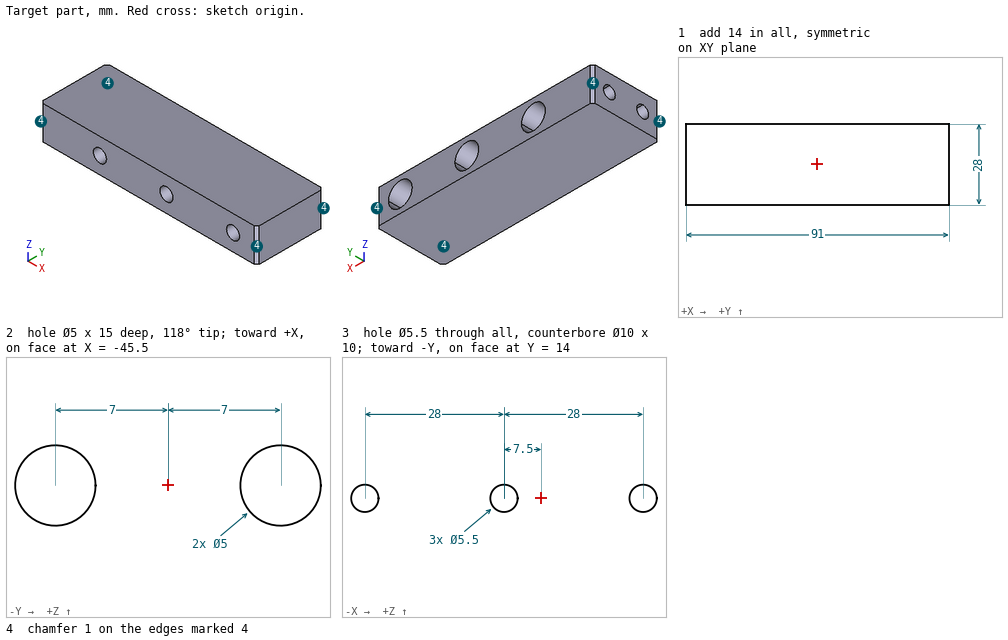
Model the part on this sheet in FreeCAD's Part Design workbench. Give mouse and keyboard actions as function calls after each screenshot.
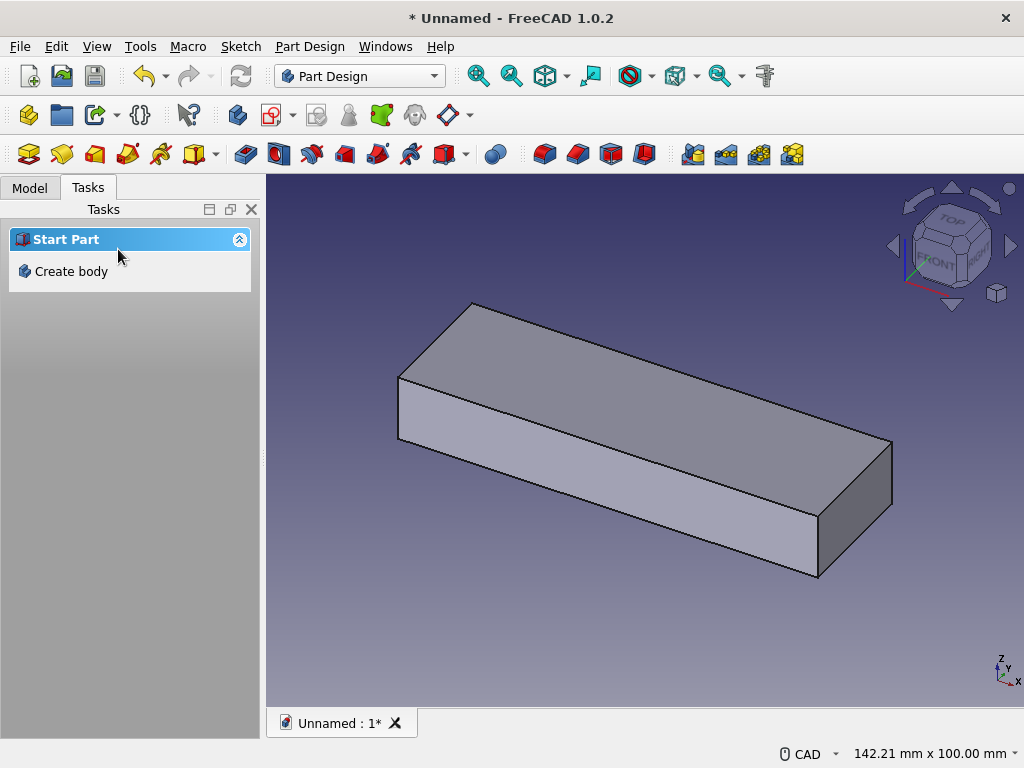
key(6)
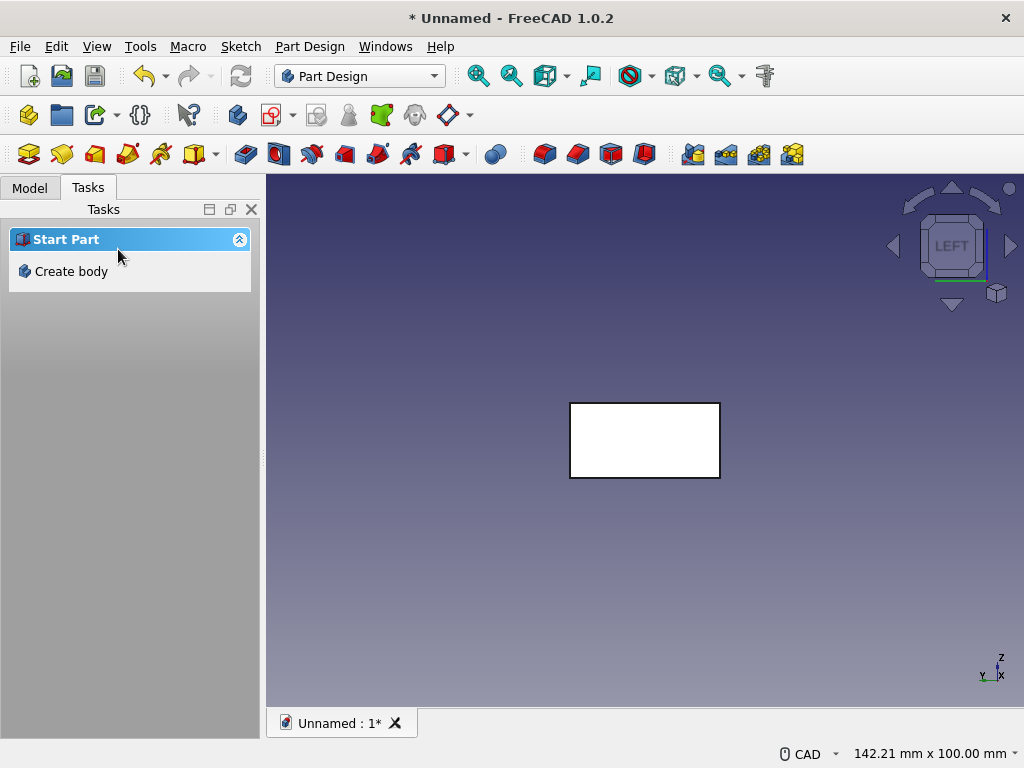
click(479, 76)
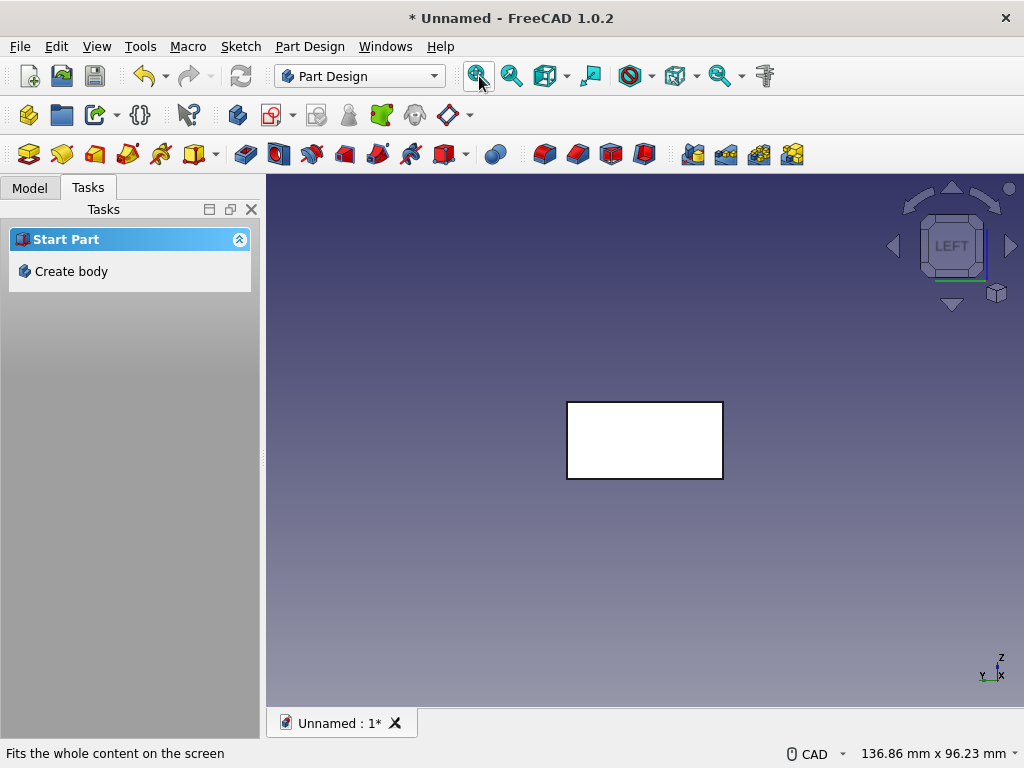
click(623, 439)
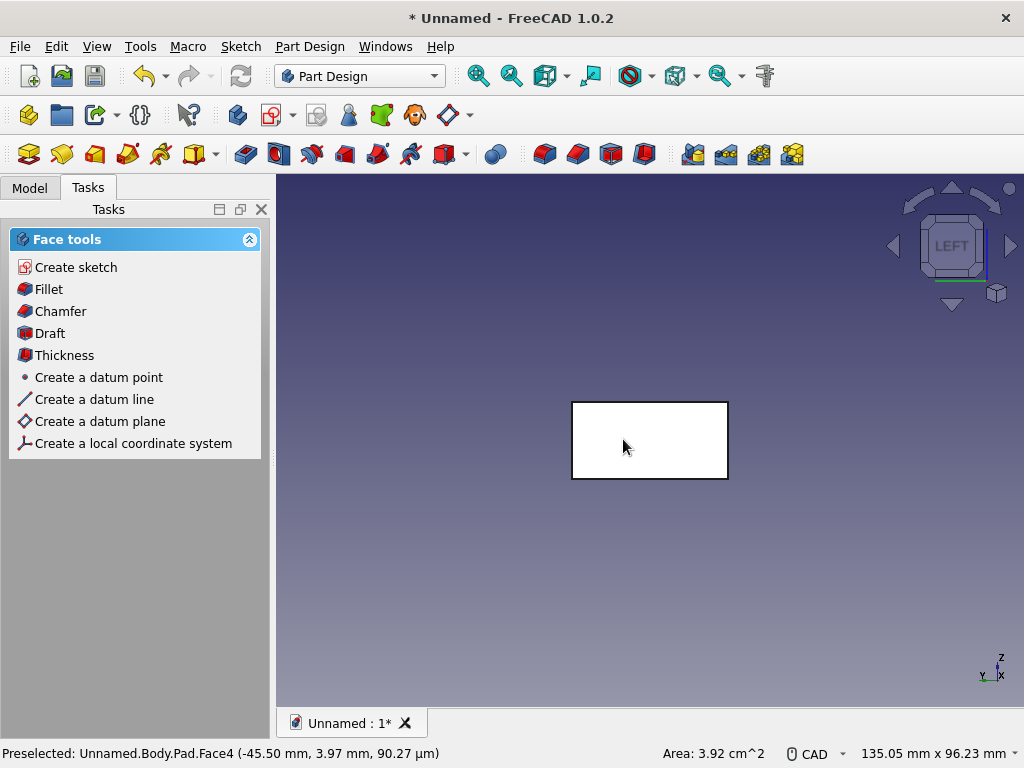
click(270, 116)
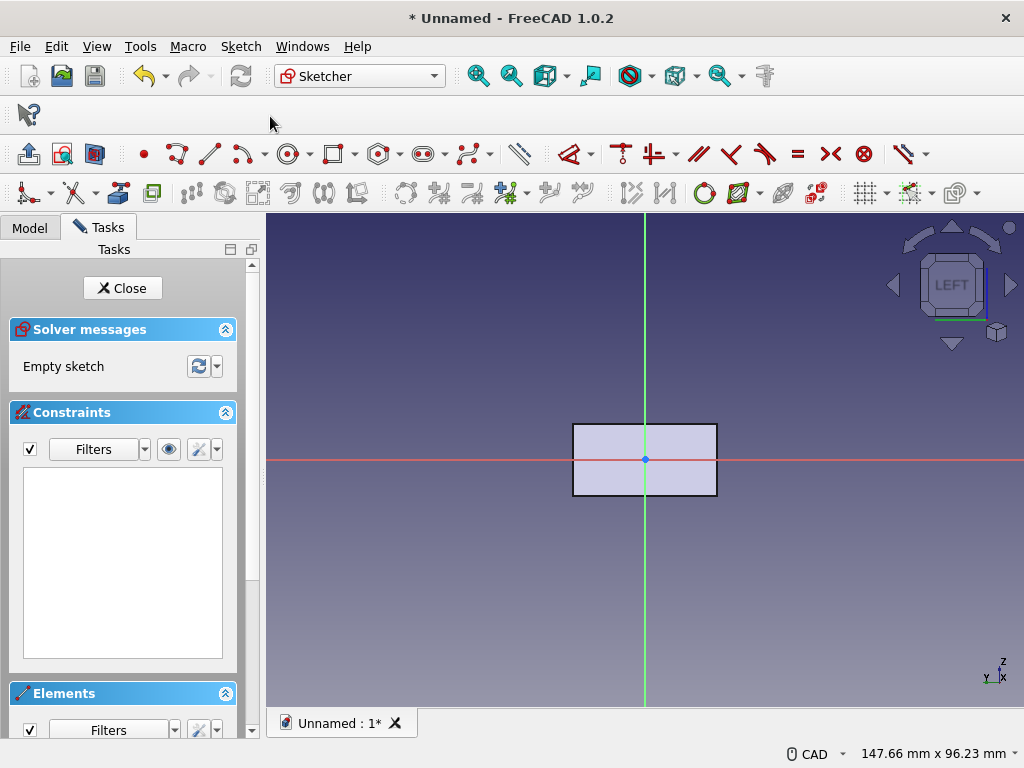
scroll(667, 460, up, 7)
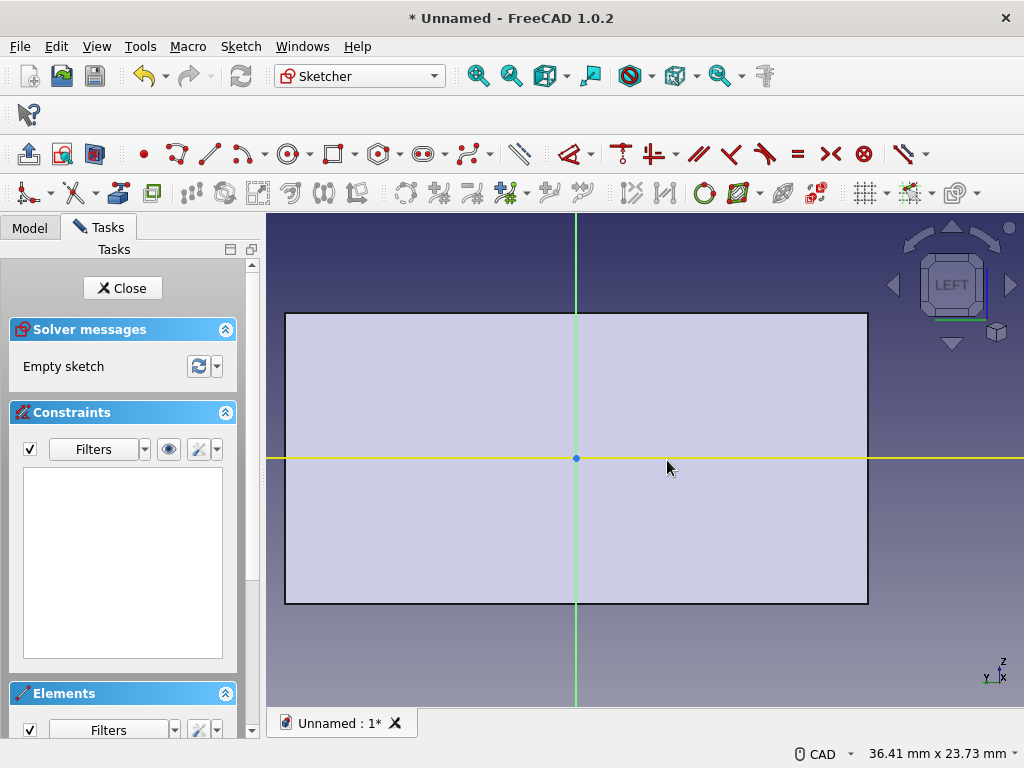
click(288, 154)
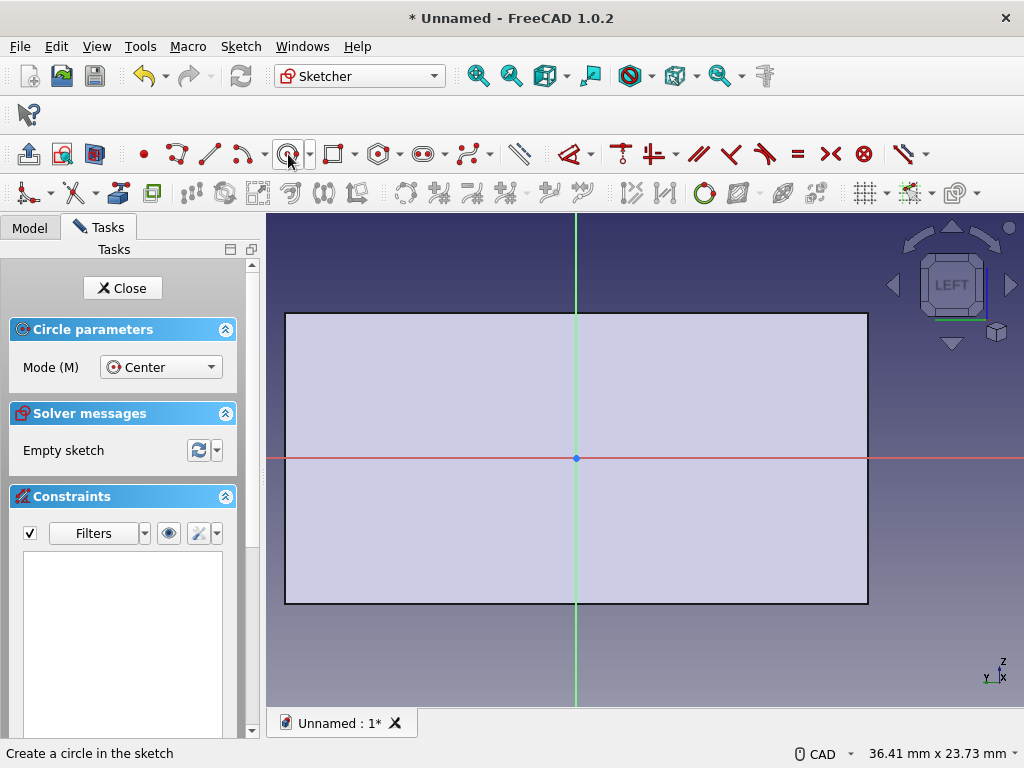
click(722, 458)
move(759, 422)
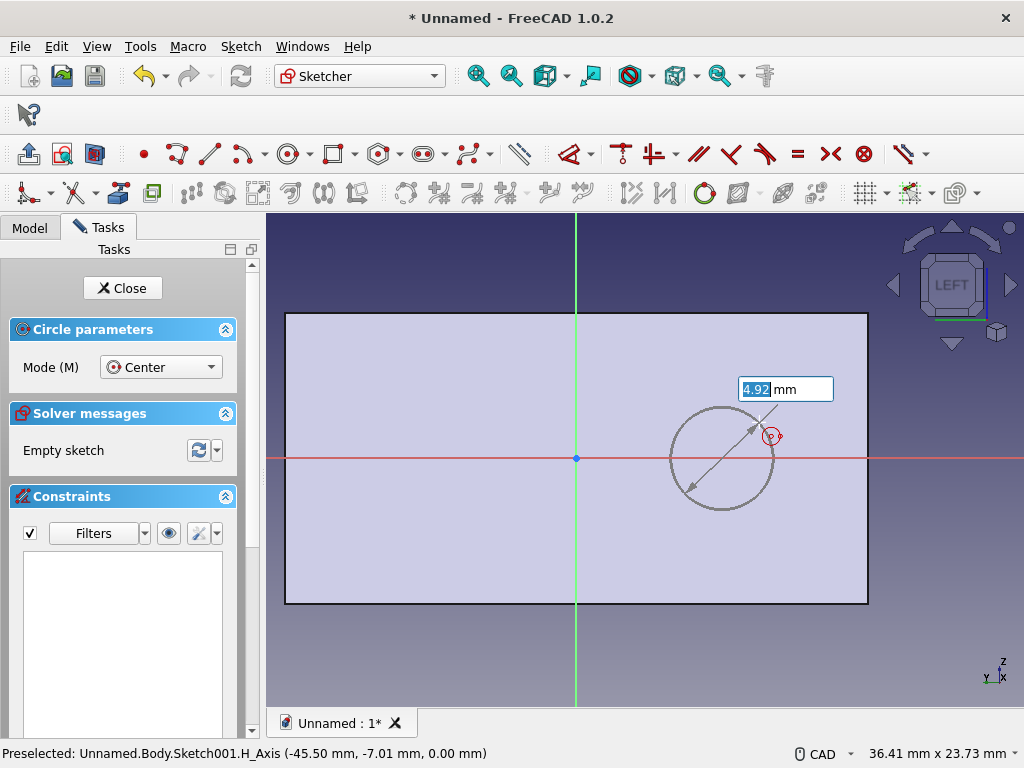
text(5)
key(Return)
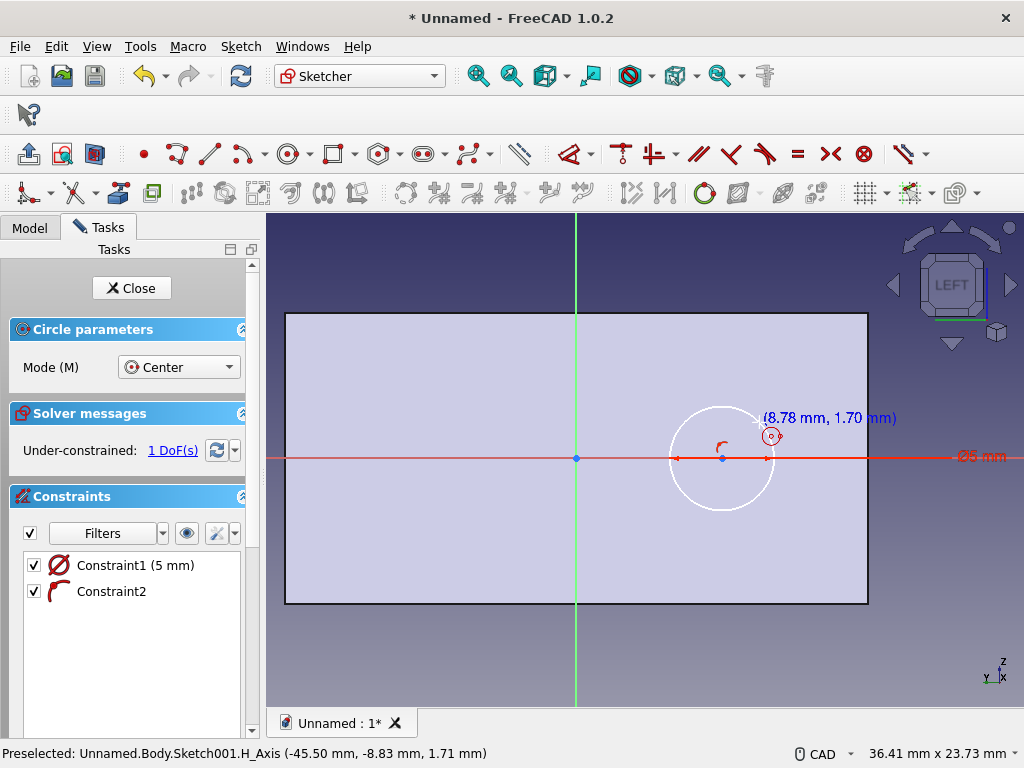
click(430, 458)
move(467, 422)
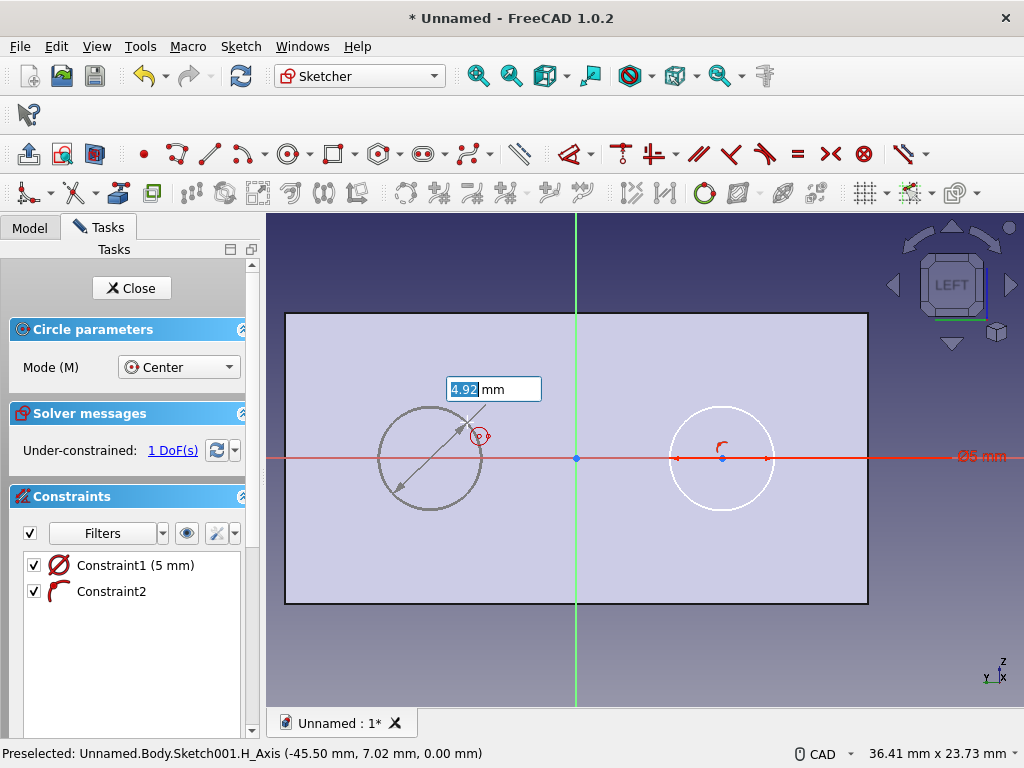
text(5)
key(Return)
key(Escape)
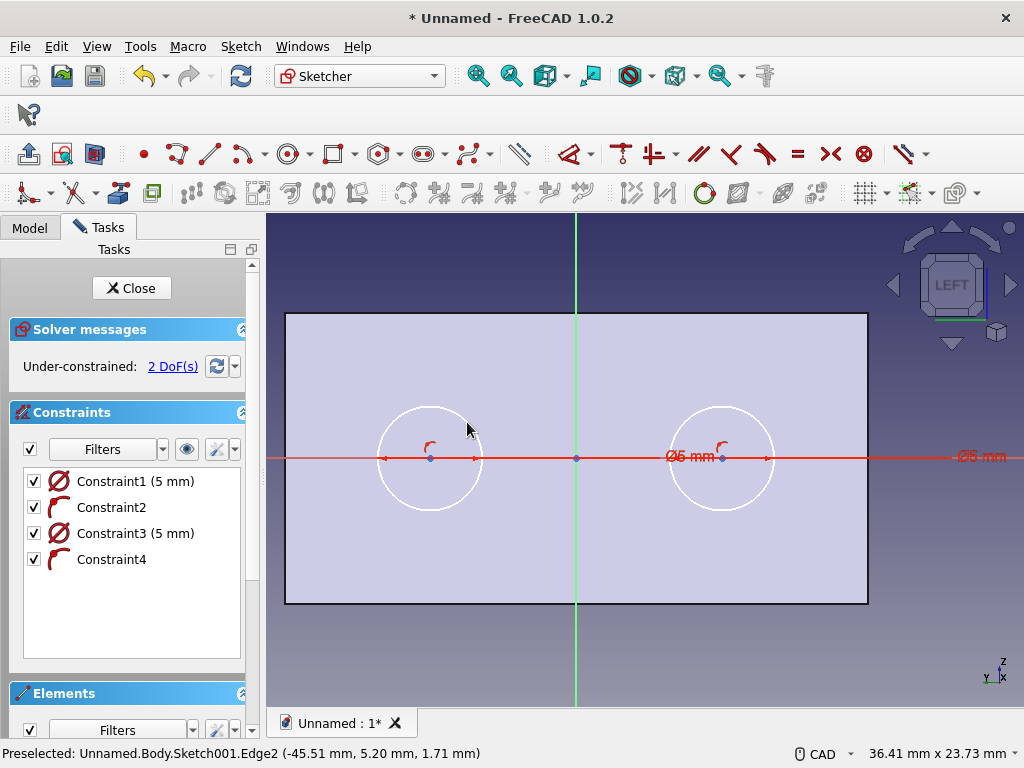
click(568, 154)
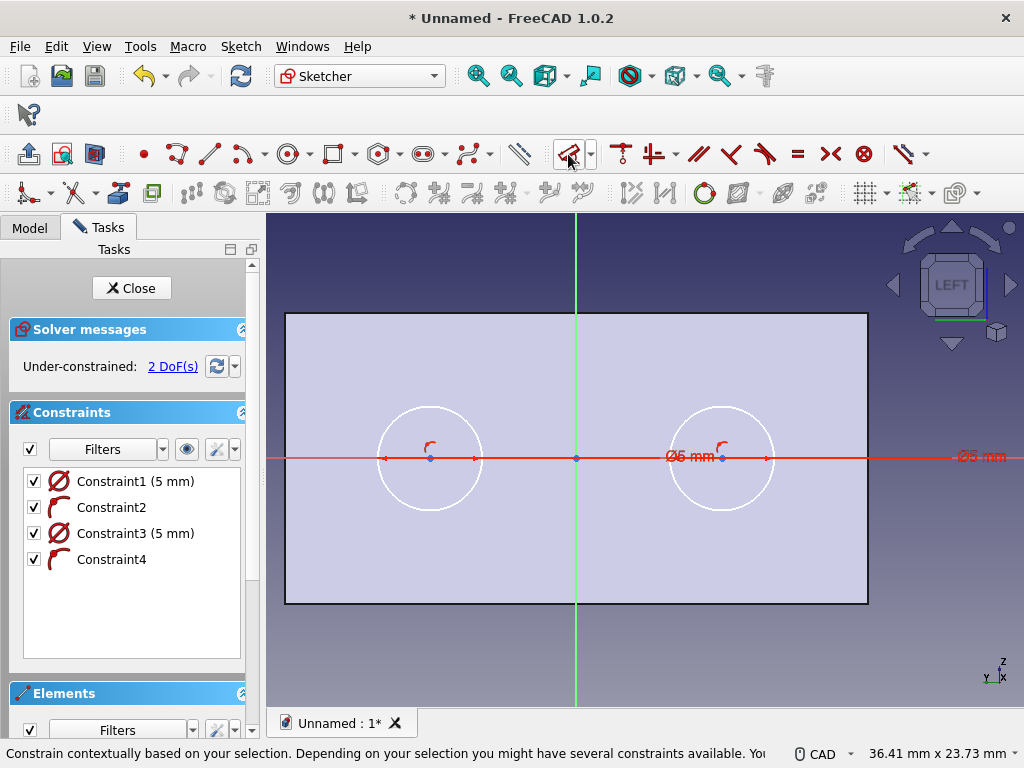
click(722, 458)
click(649, 492)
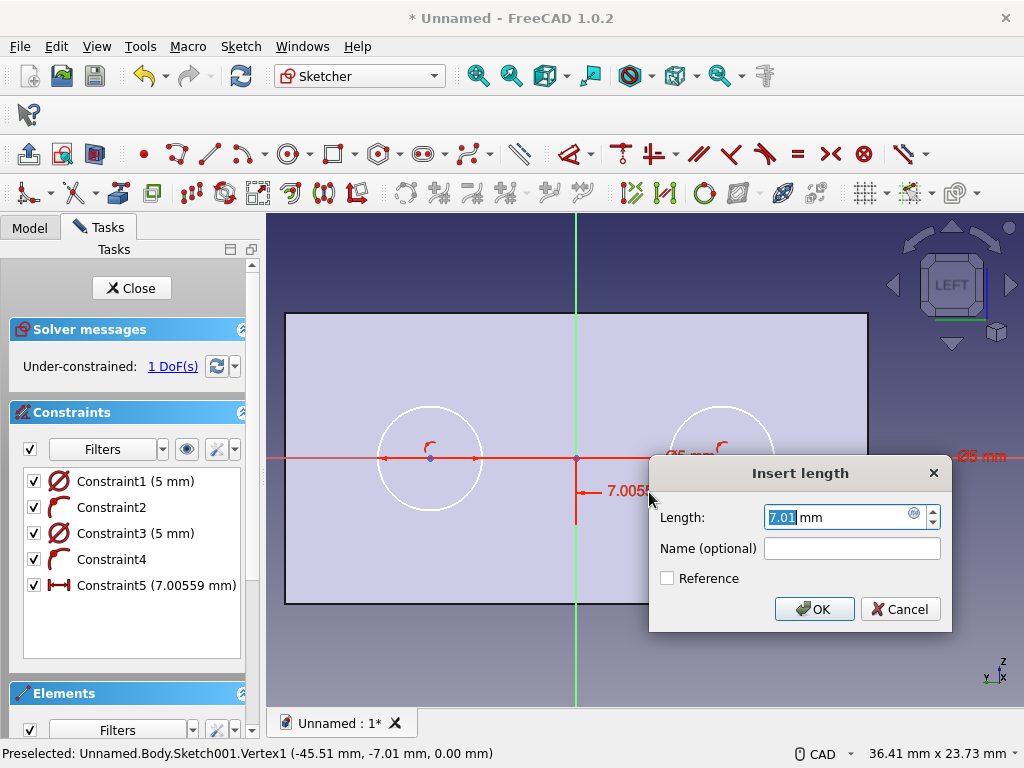
text(7)
key(Return)